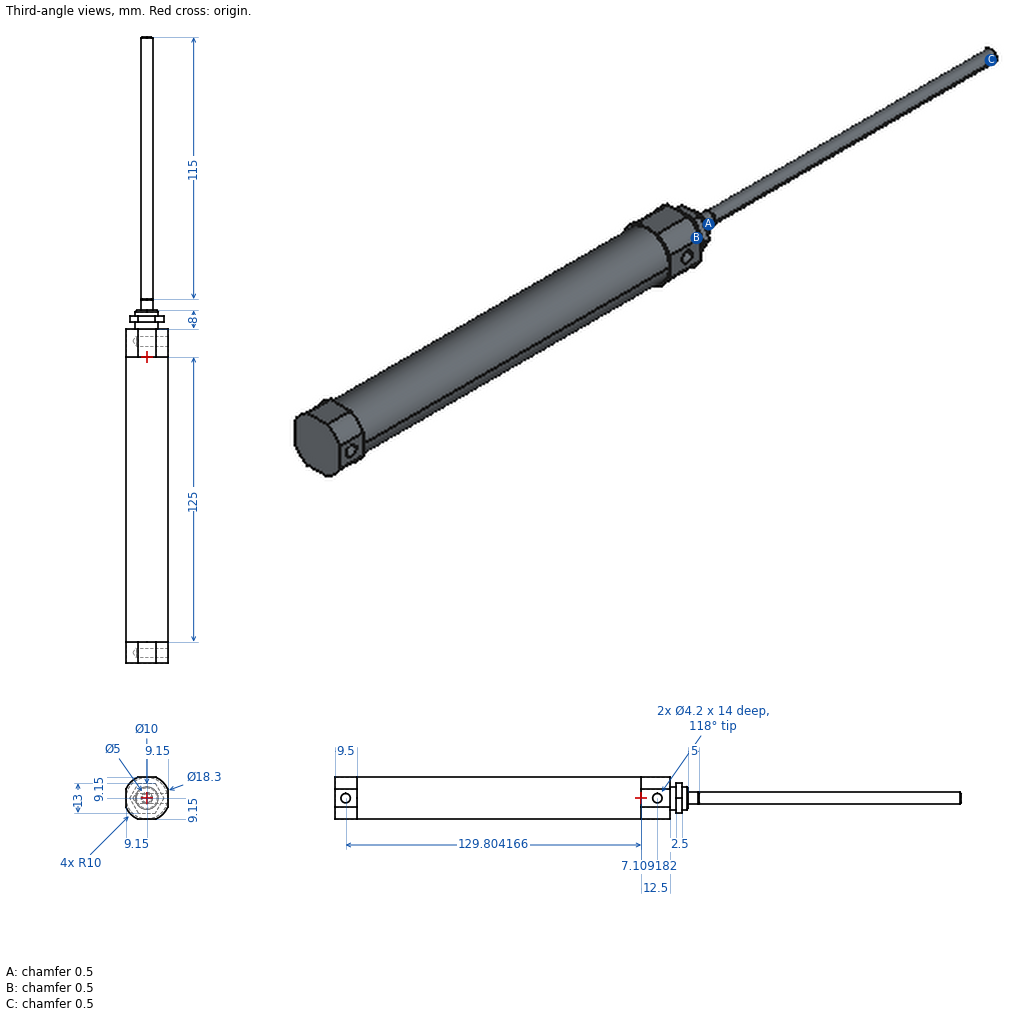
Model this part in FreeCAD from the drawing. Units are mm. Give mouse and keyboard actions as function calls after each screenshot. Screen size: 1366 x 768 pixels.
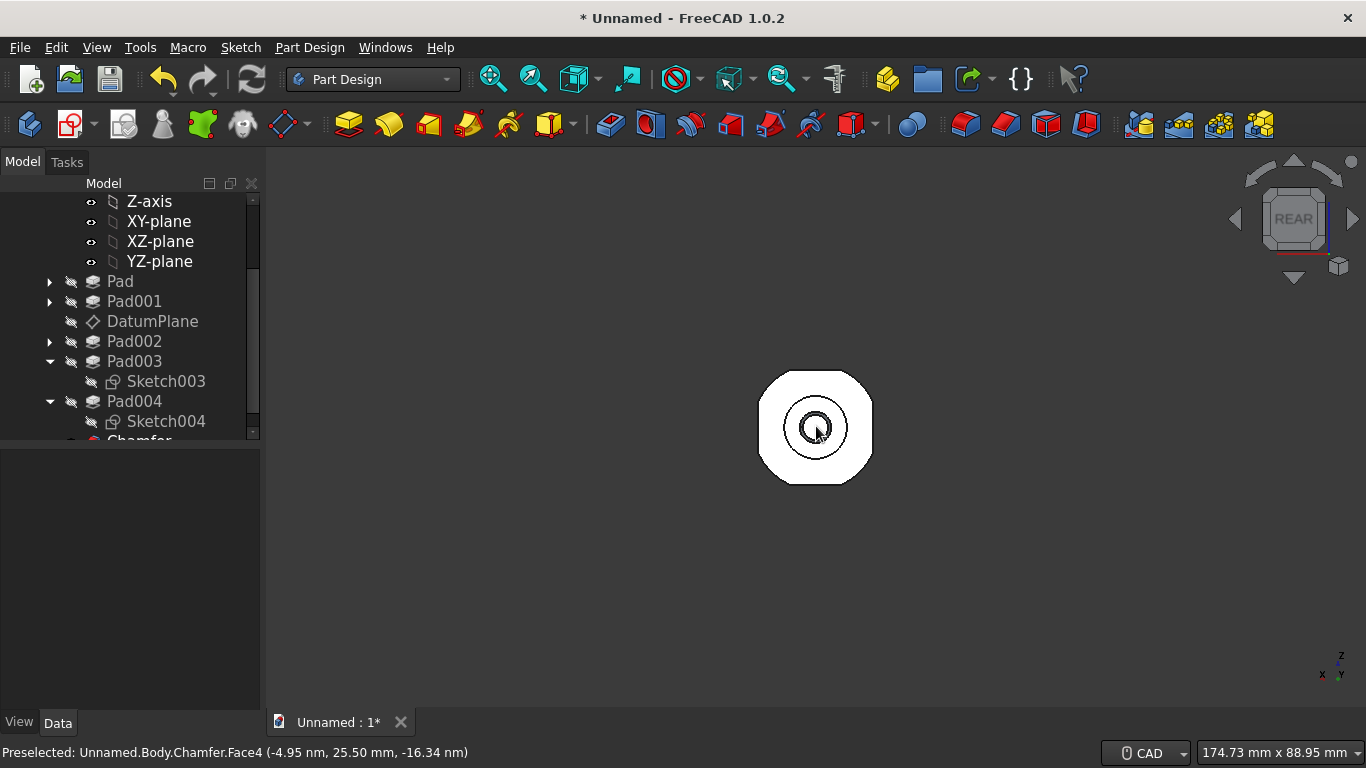
click(816, 426)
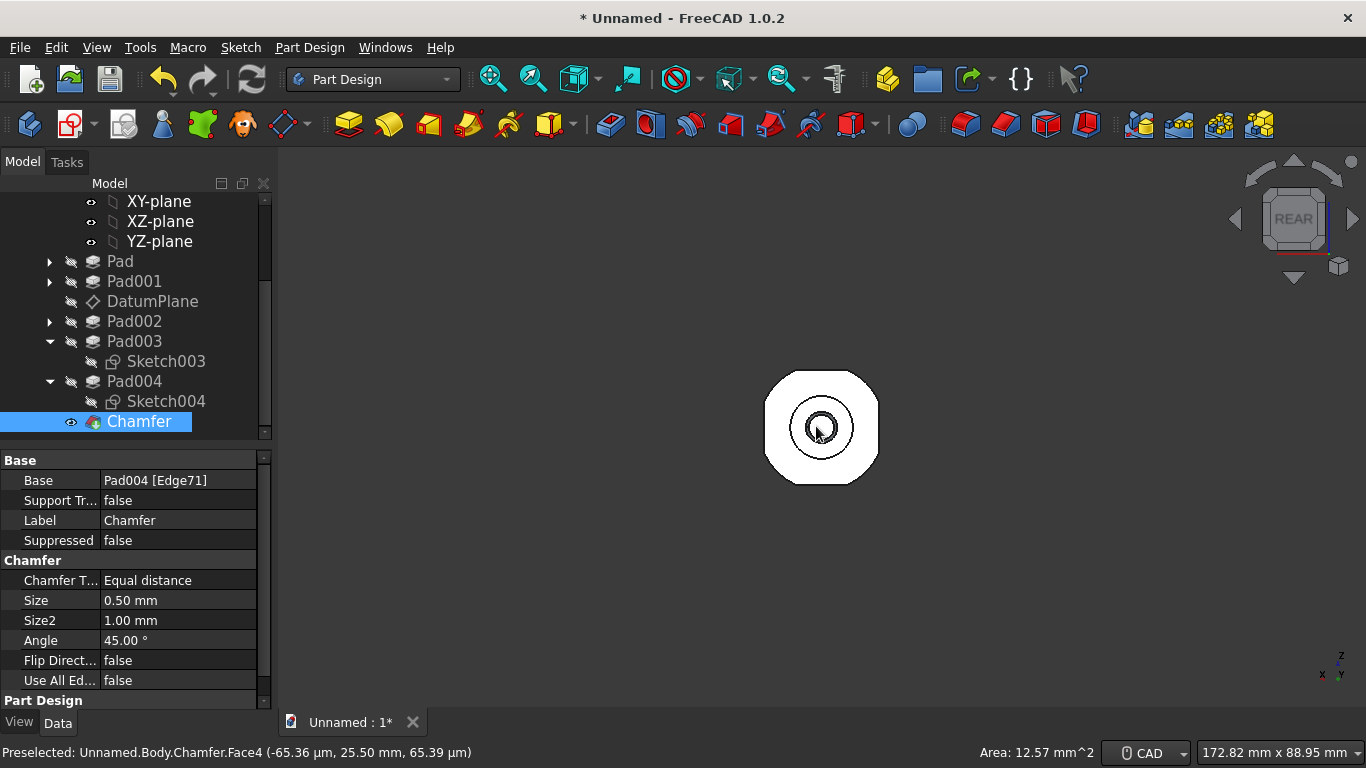
click(70, 124)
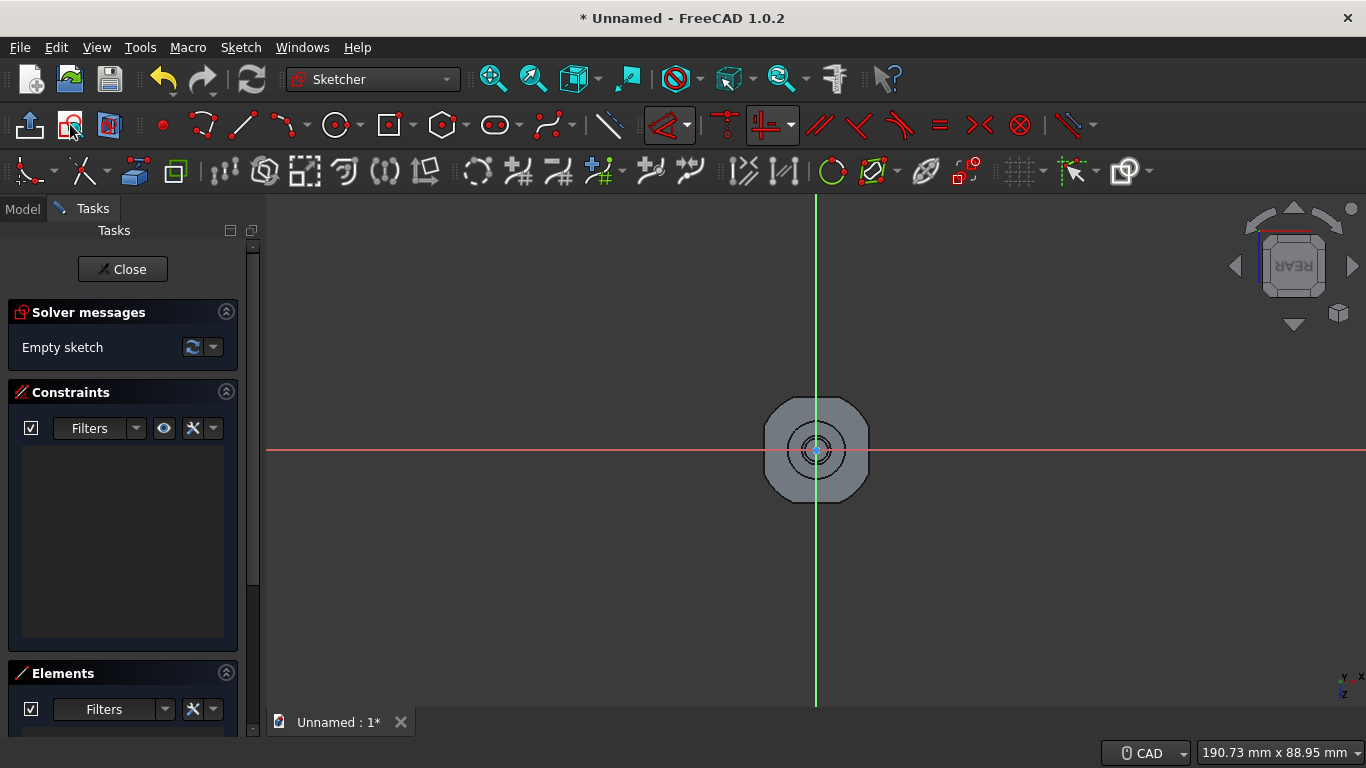
scroll(823, 450, up, 12)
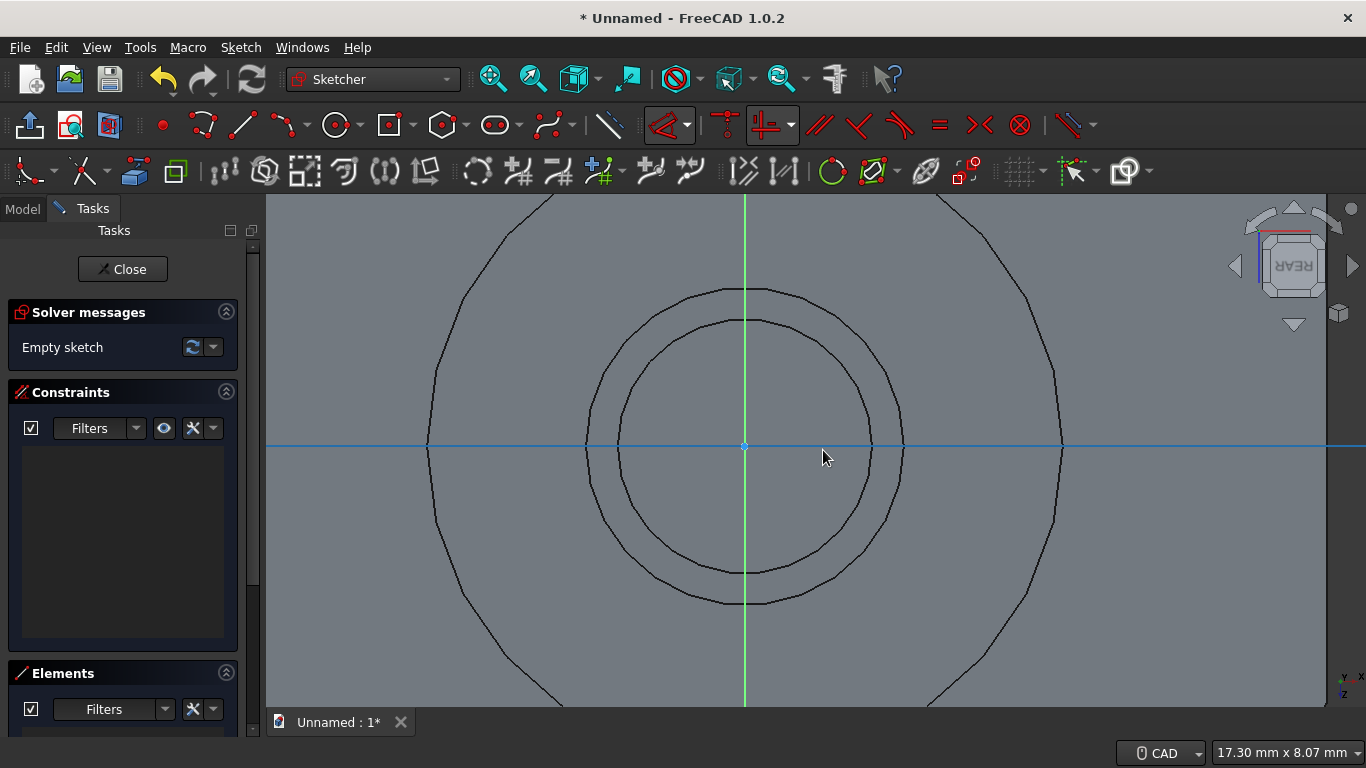
click(336, 126)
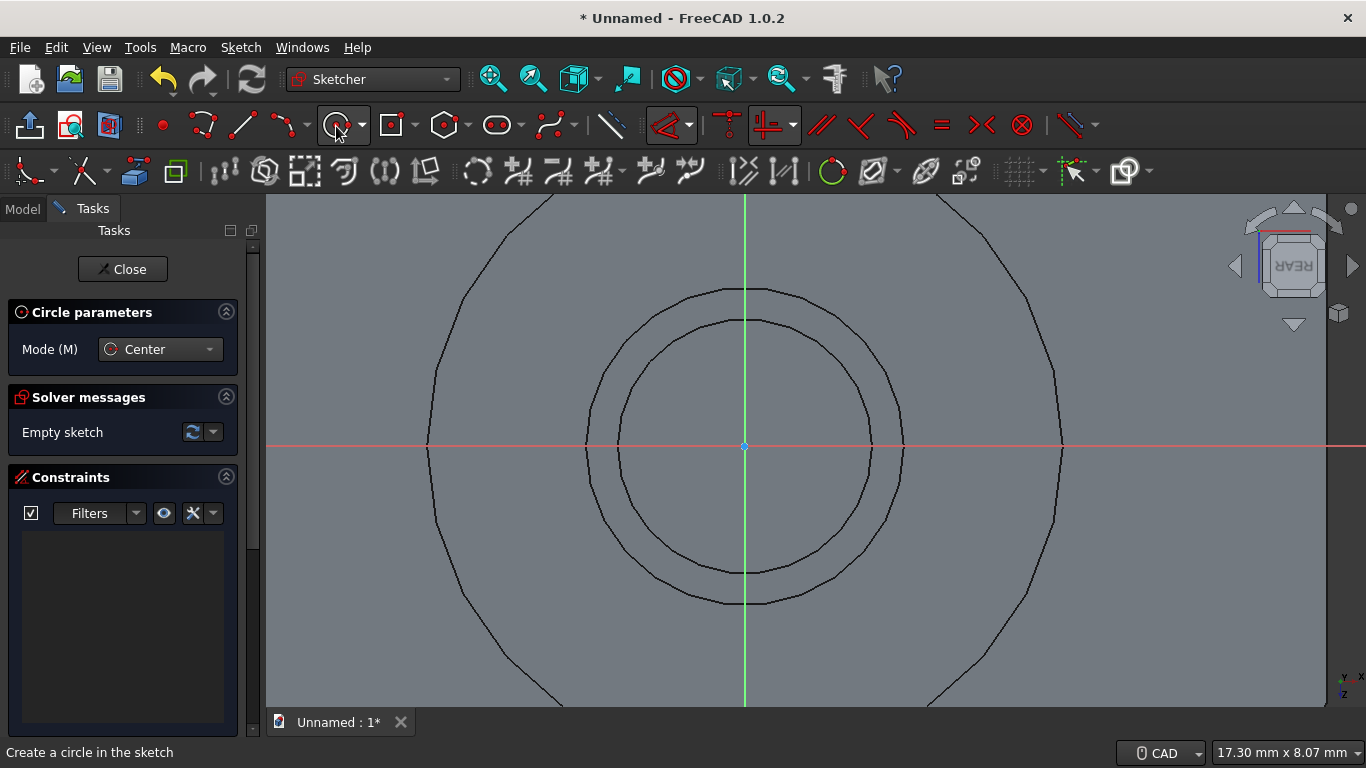
click(745, 446)
click(857, 334)
key(Escape)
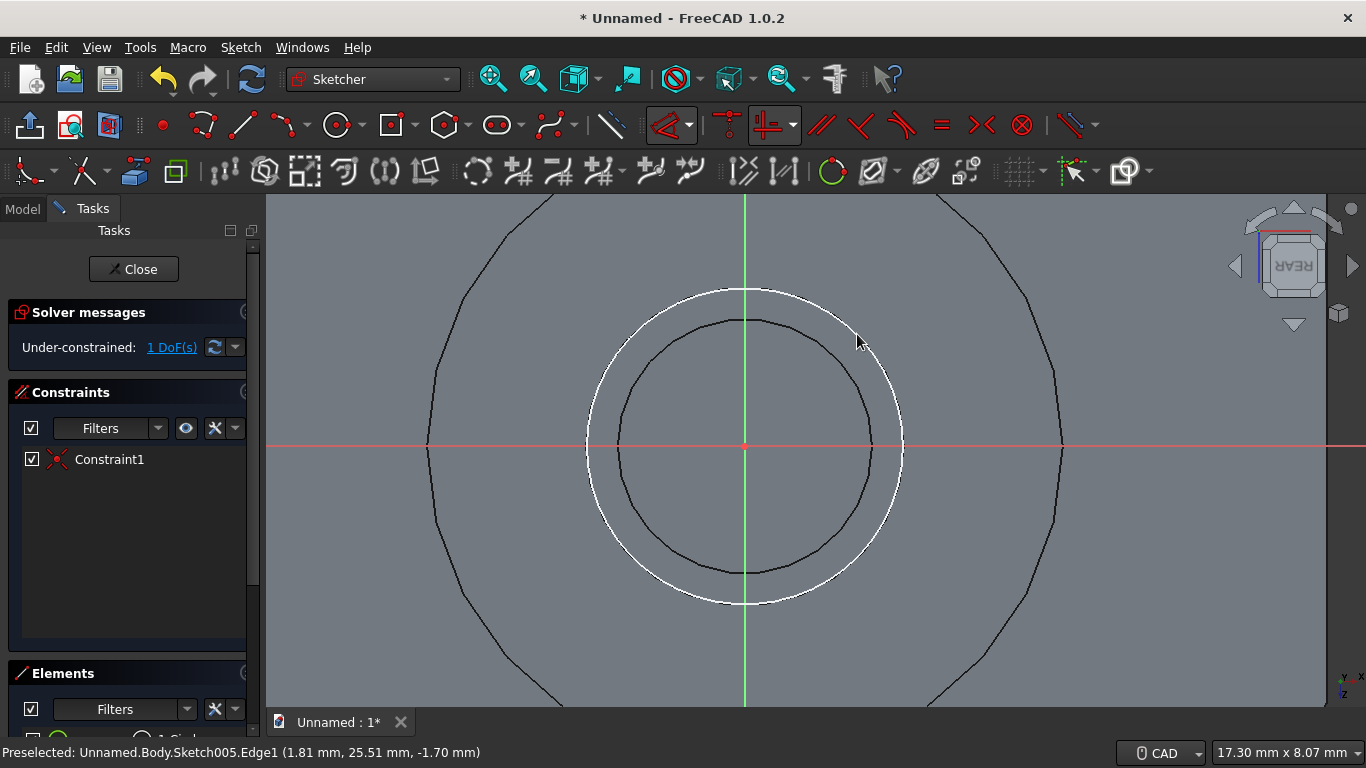
click(666, 126)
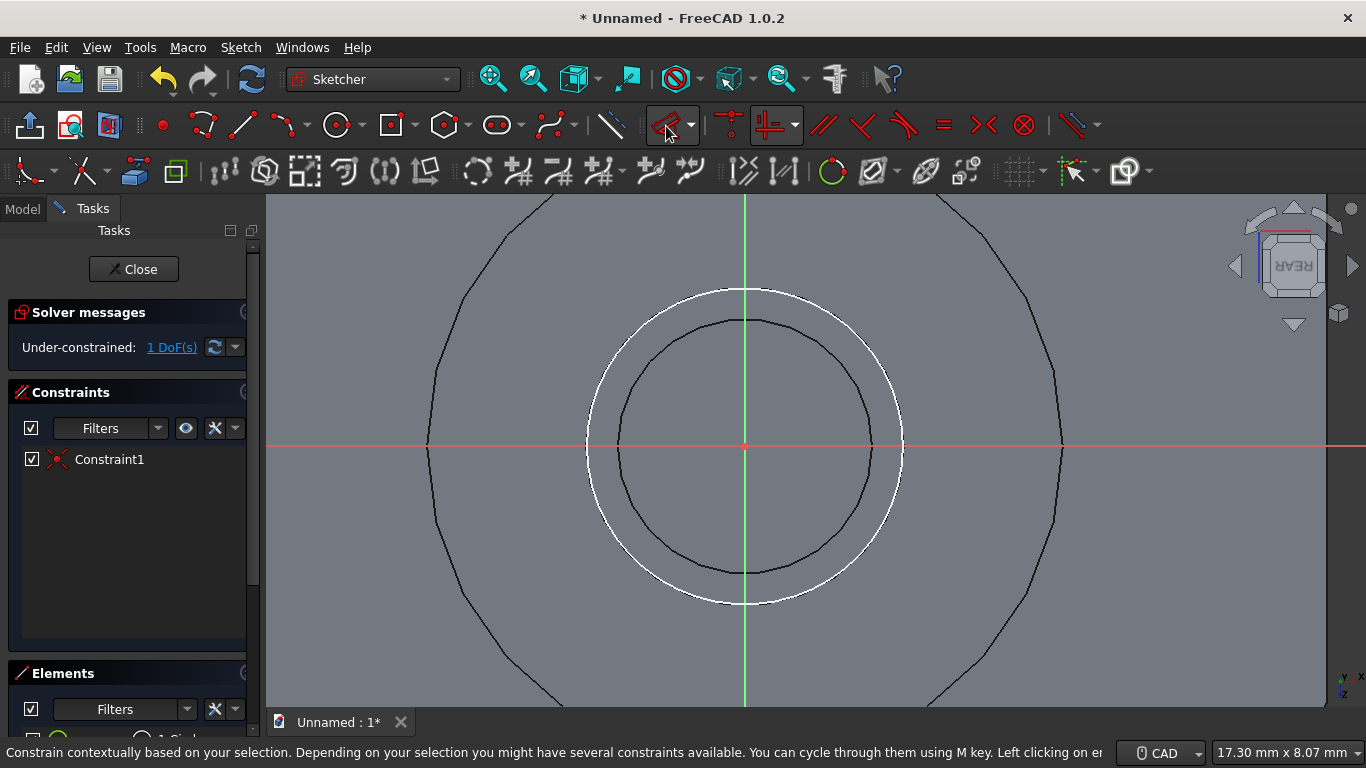
click(856, 334)
click(878, 311)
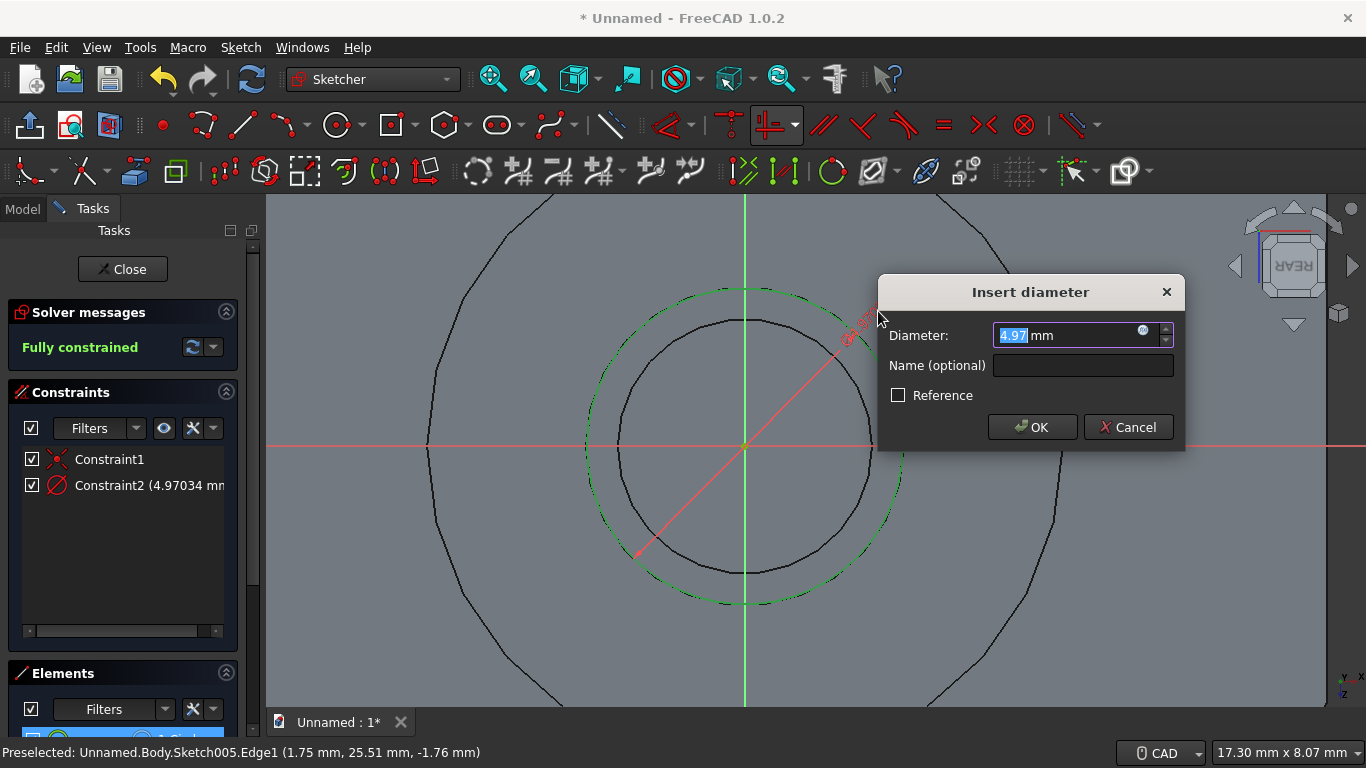
text(5)
key(Return)
key(Escape)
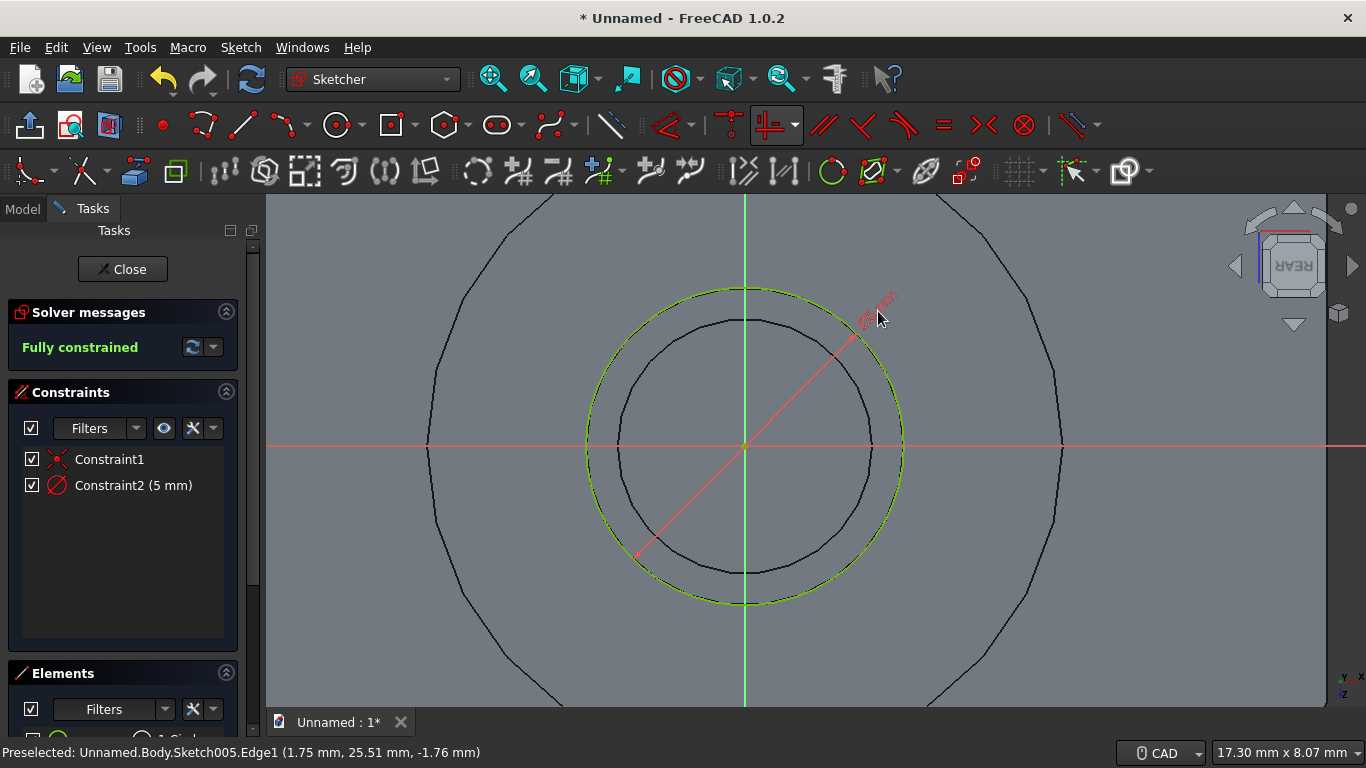
click(123, 269)